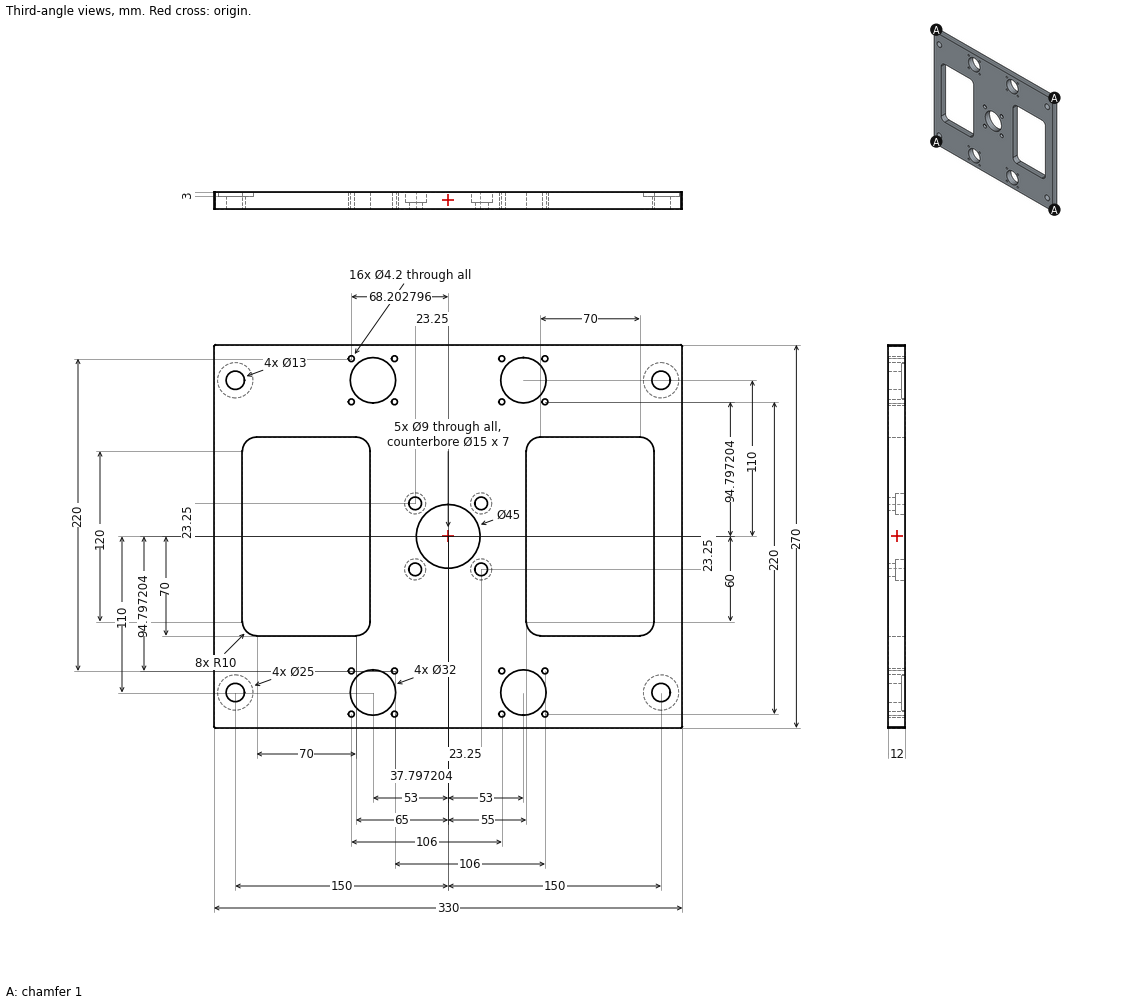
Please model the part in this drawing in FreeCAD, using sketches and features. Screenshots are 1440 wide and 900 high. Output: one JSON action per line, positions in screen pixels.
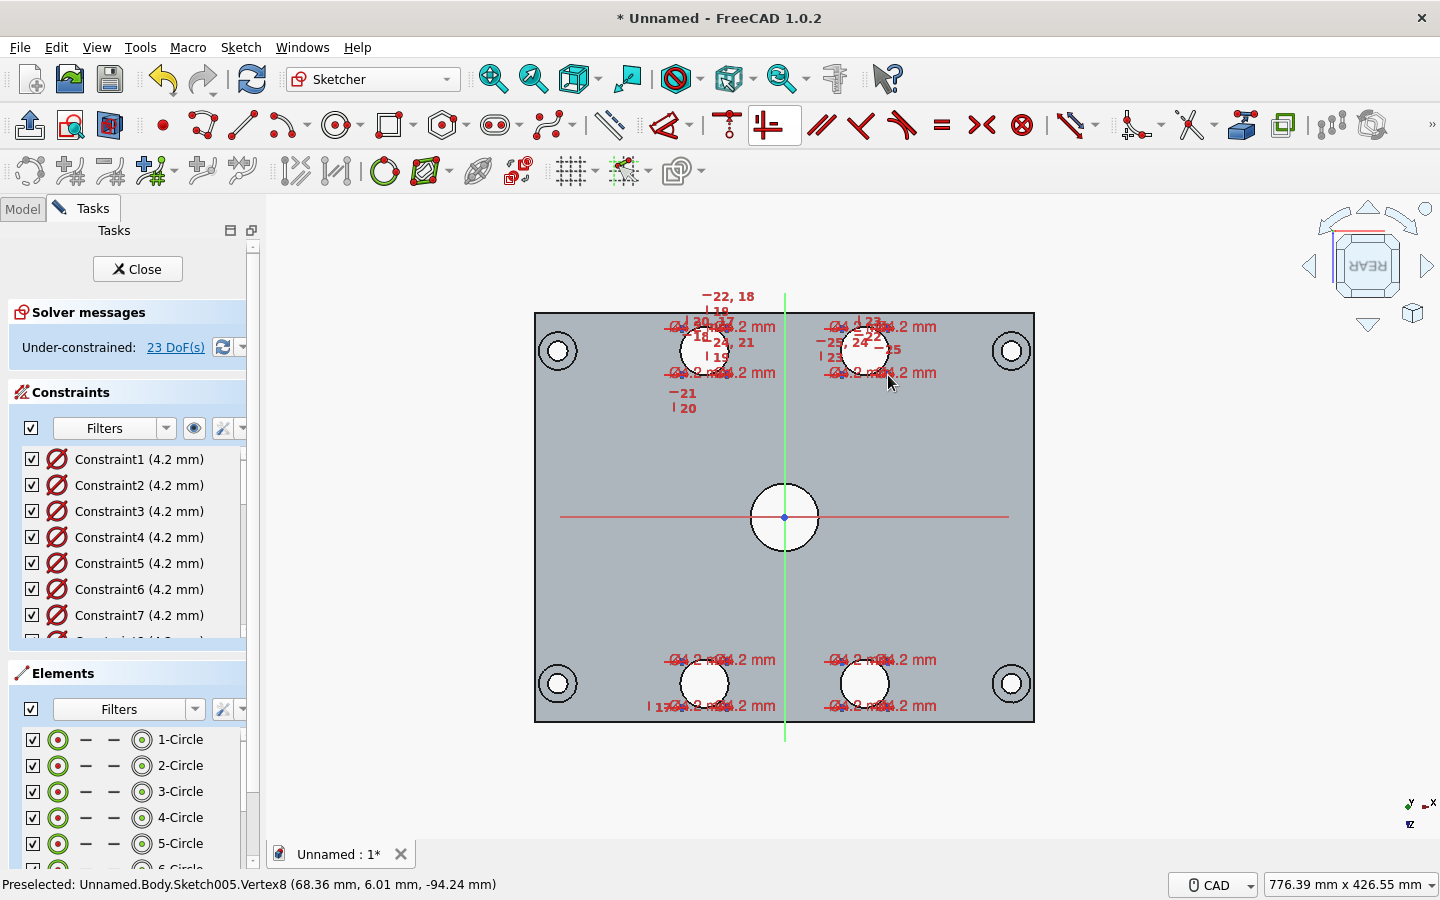
{"action": "left_click", "coordinate": [888, 375]}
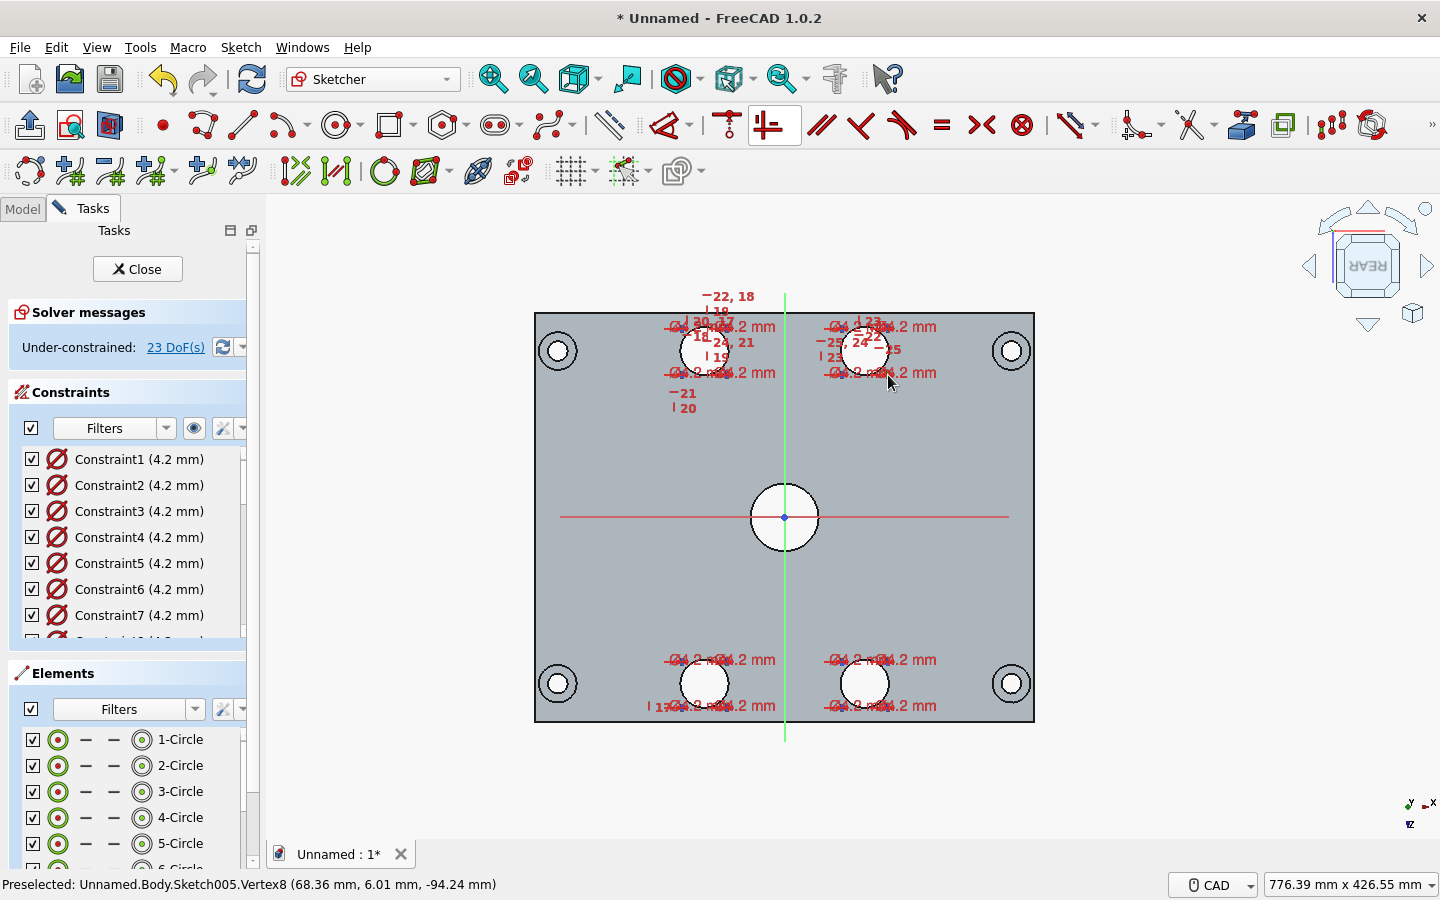
{"action": "left_click", "coordinate": [888, 329]}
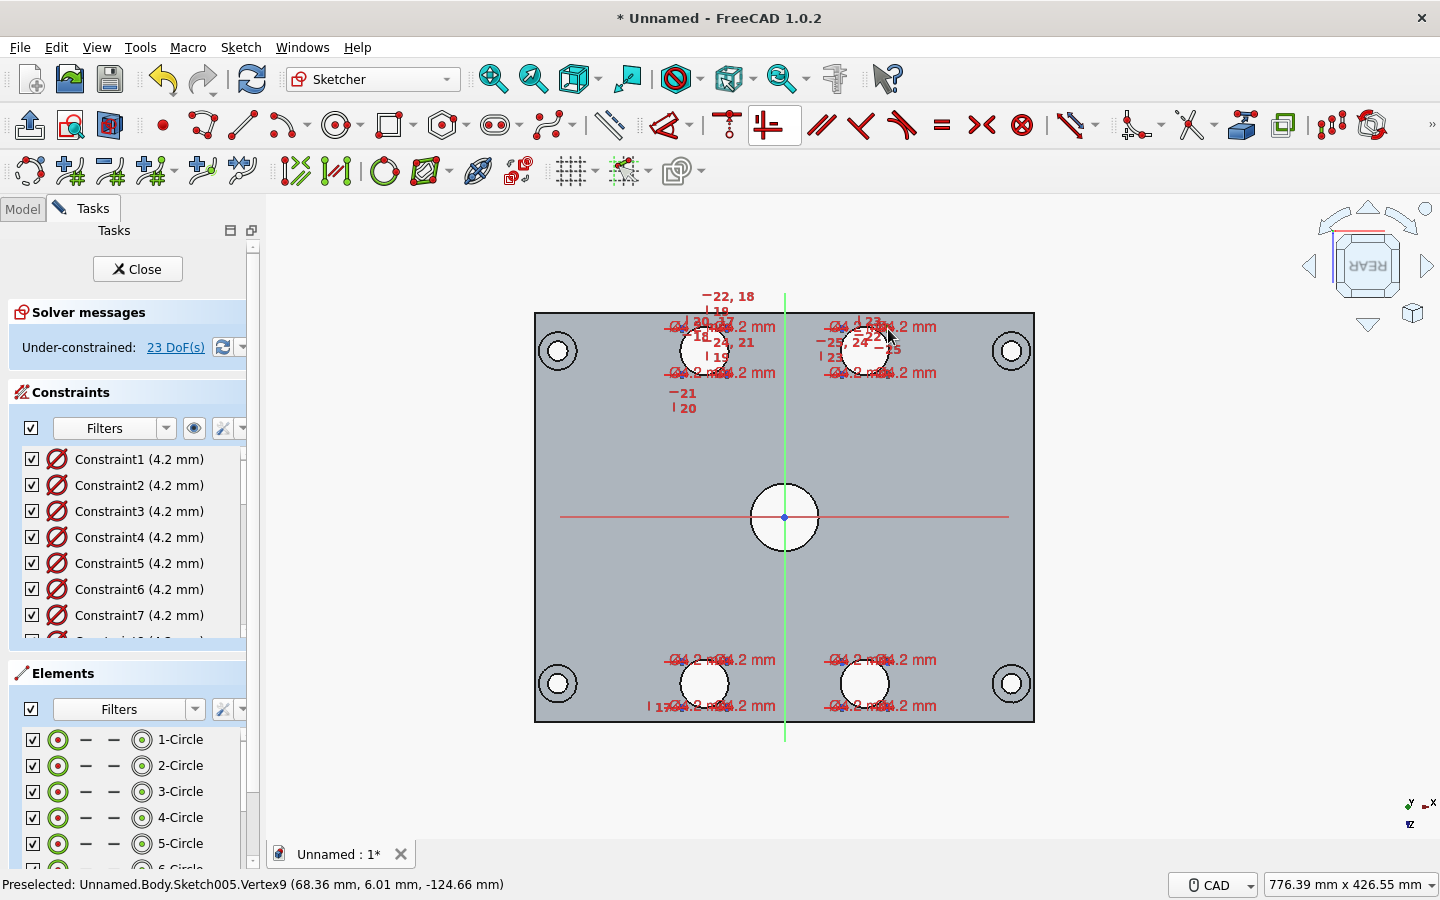
{"action": "left_click", "coordinate": [796, 126]}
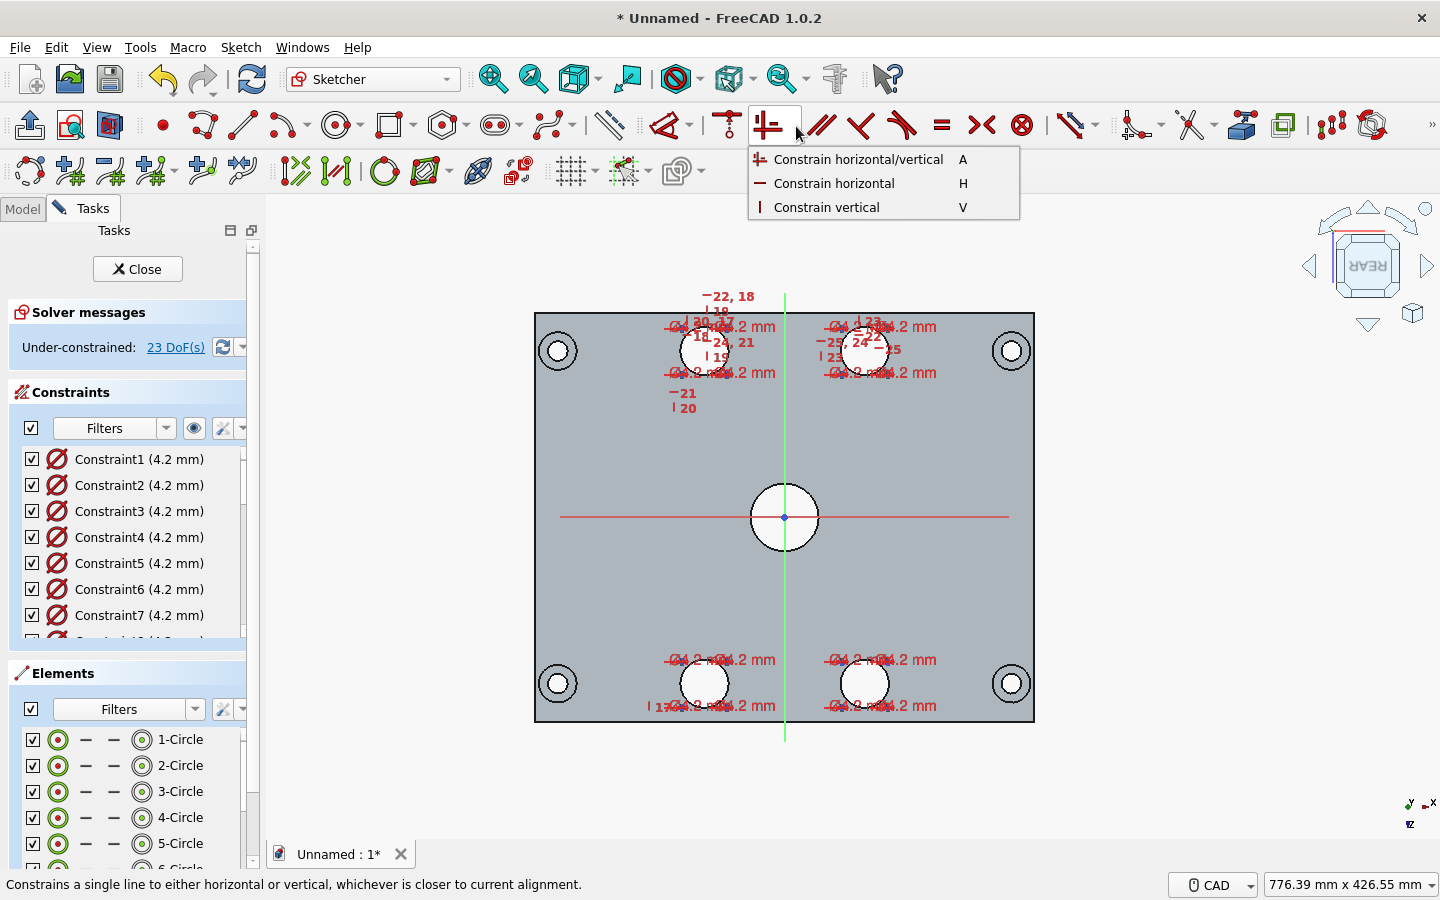
{"action": "left_click", "coordinate": [884, 207]}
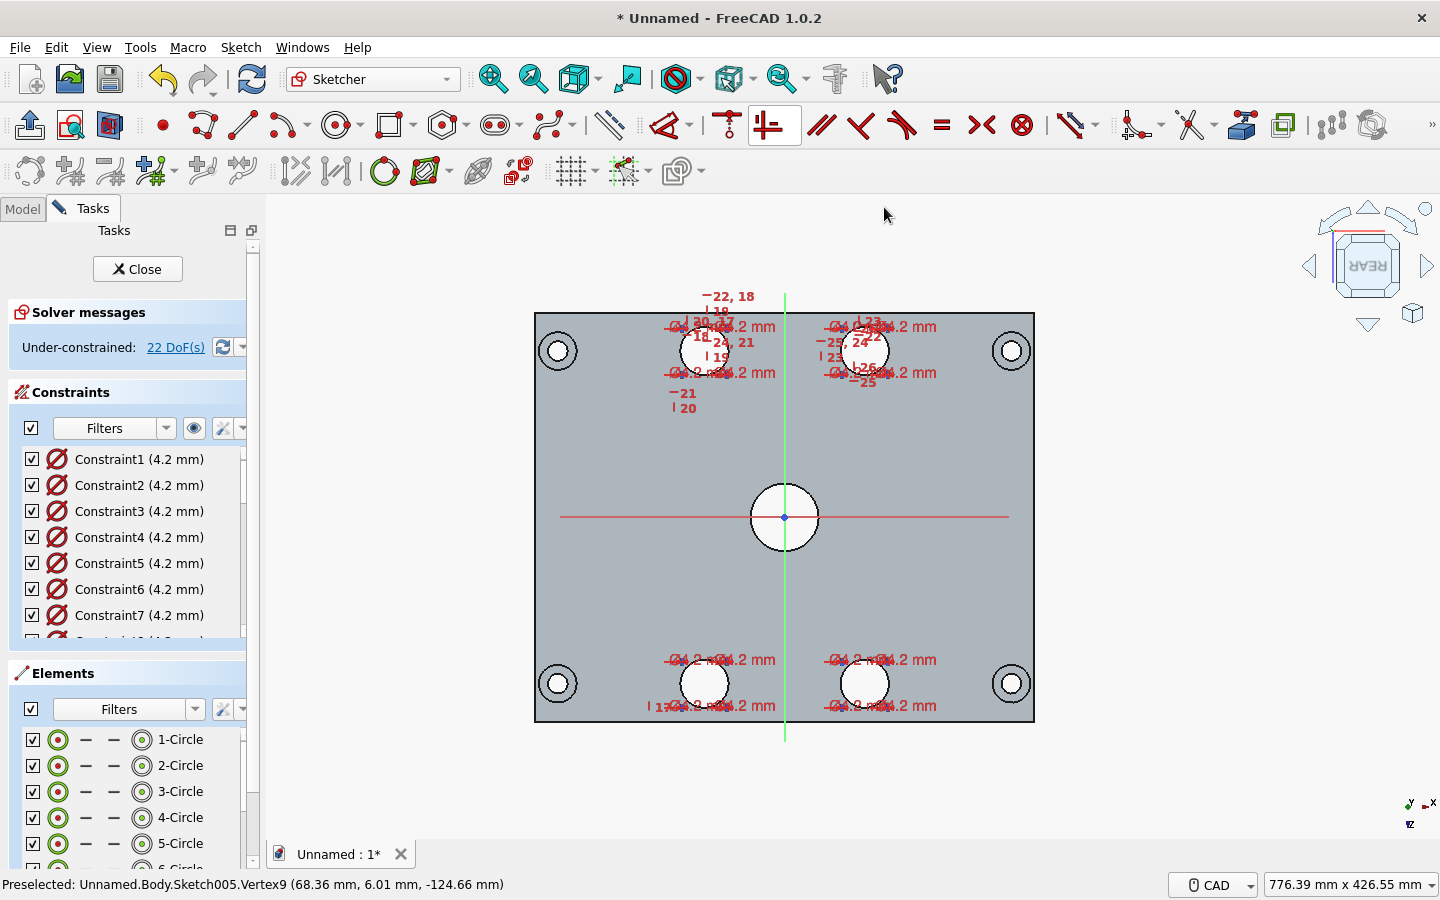
{"action": "left_click", "coordinate": [842, 329]}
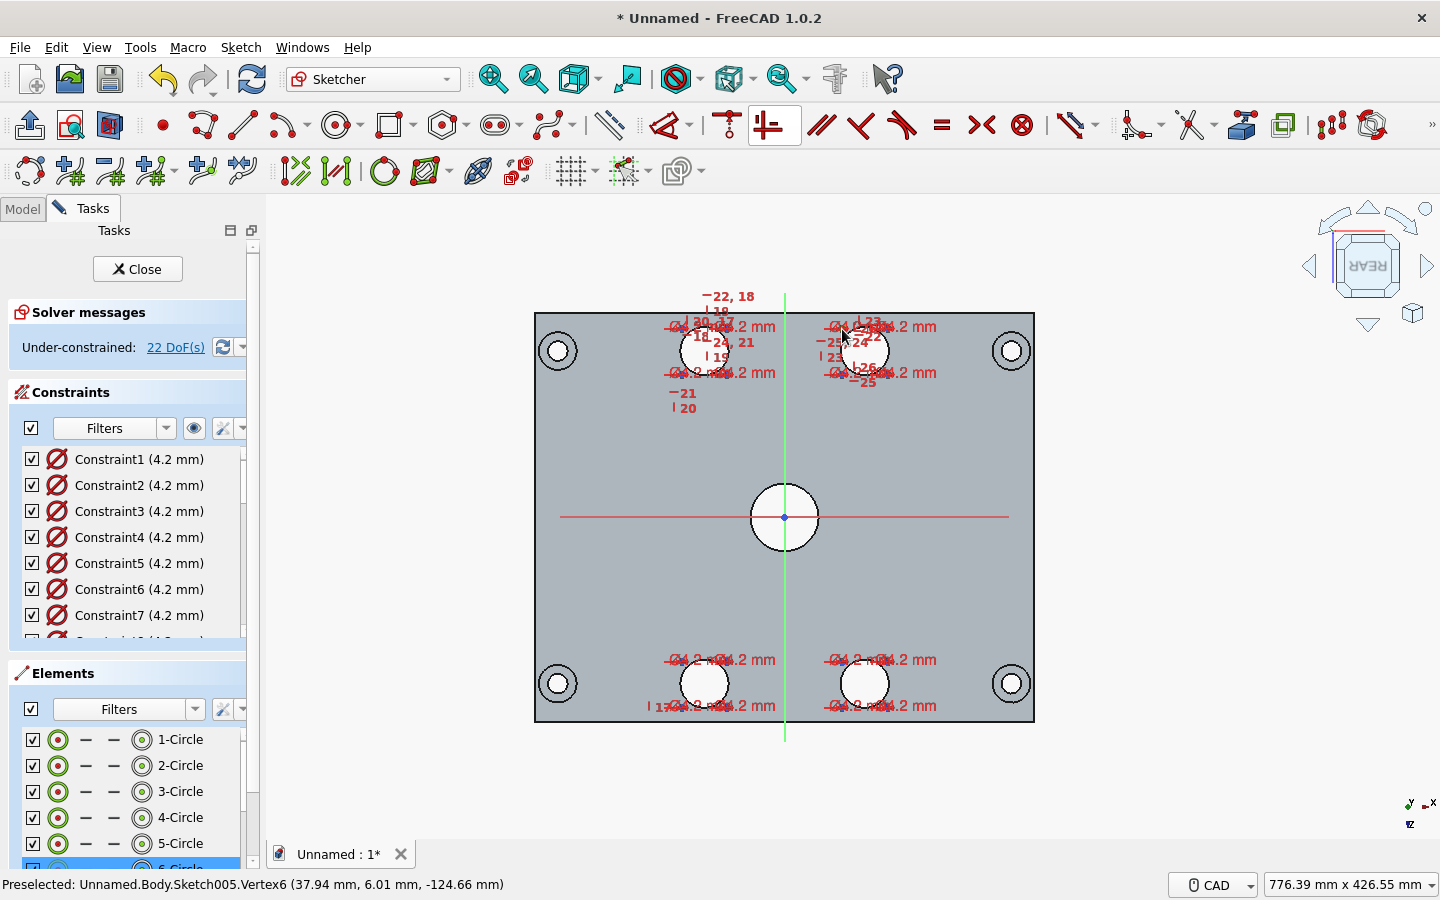
{"action": "left_click", "coordinate": [888, 329]}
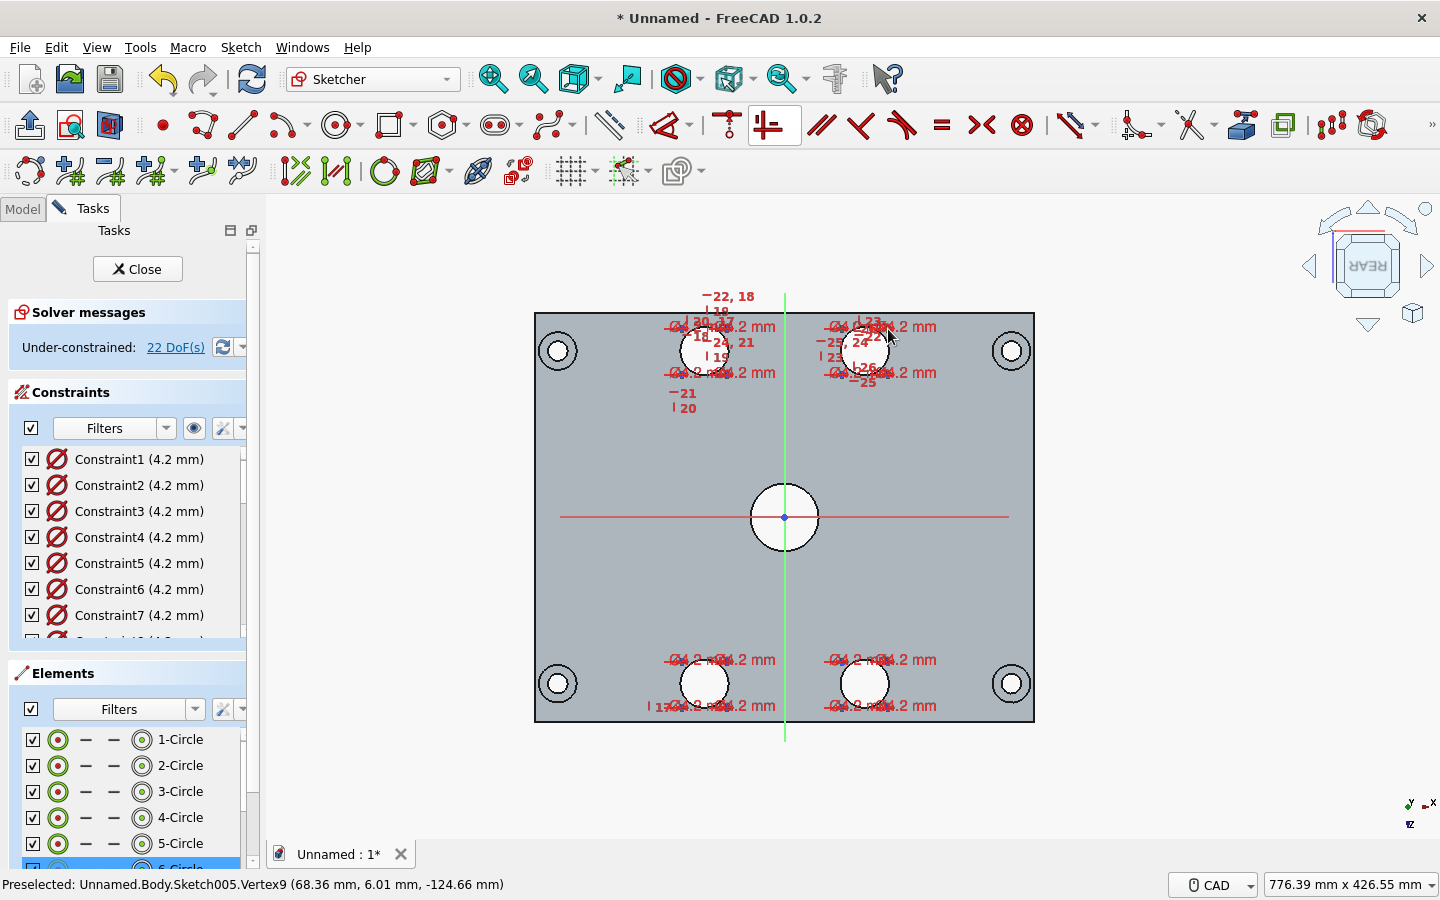
{"action": "left_click", "coordinate": [796, 126]}